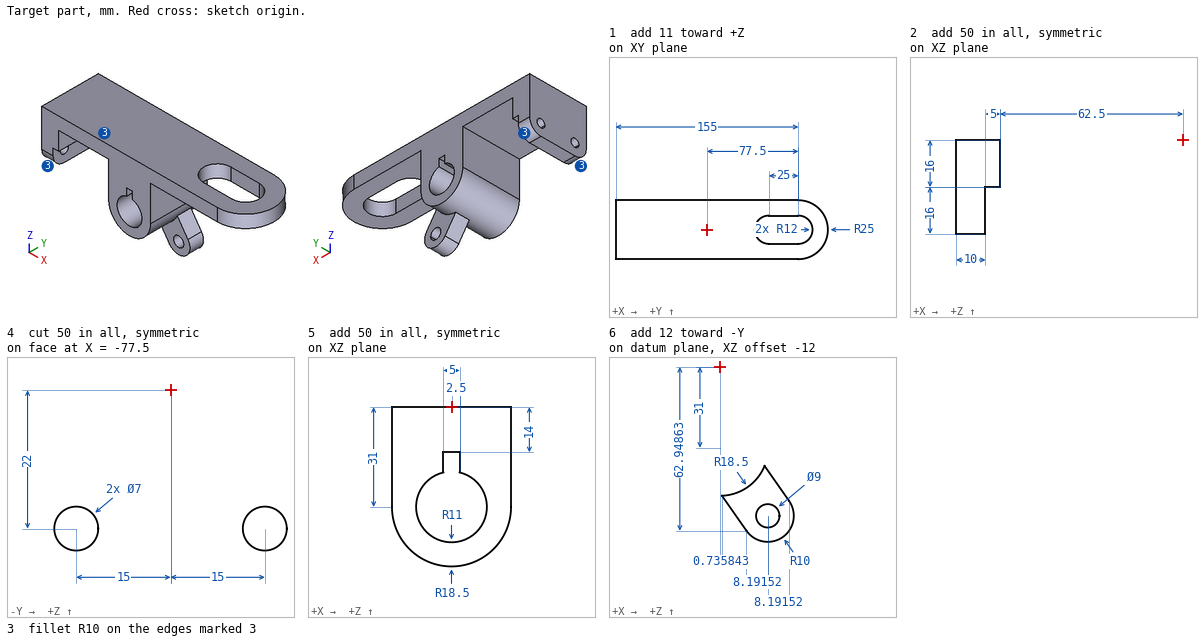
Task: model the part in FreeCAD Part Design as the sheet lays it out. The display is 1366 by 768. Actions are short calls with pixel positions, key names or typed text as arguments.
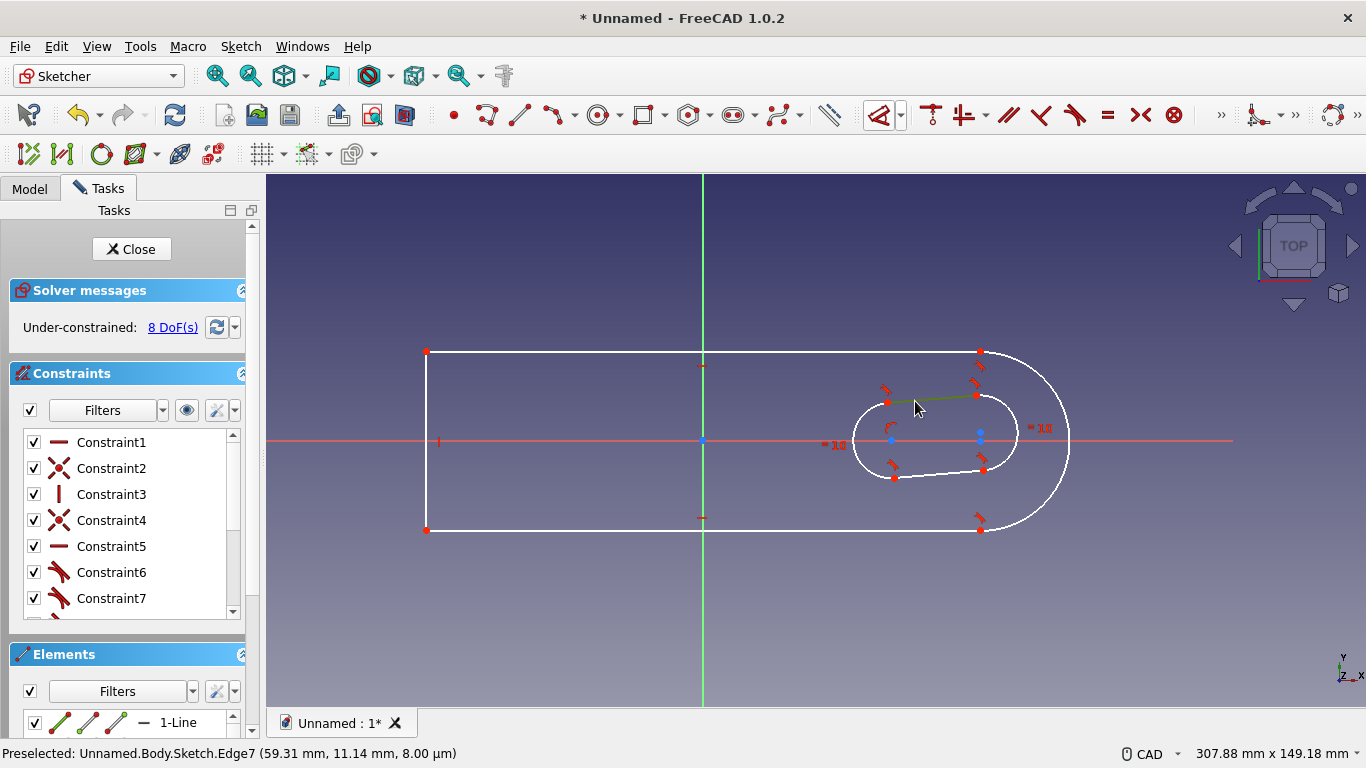
key(h)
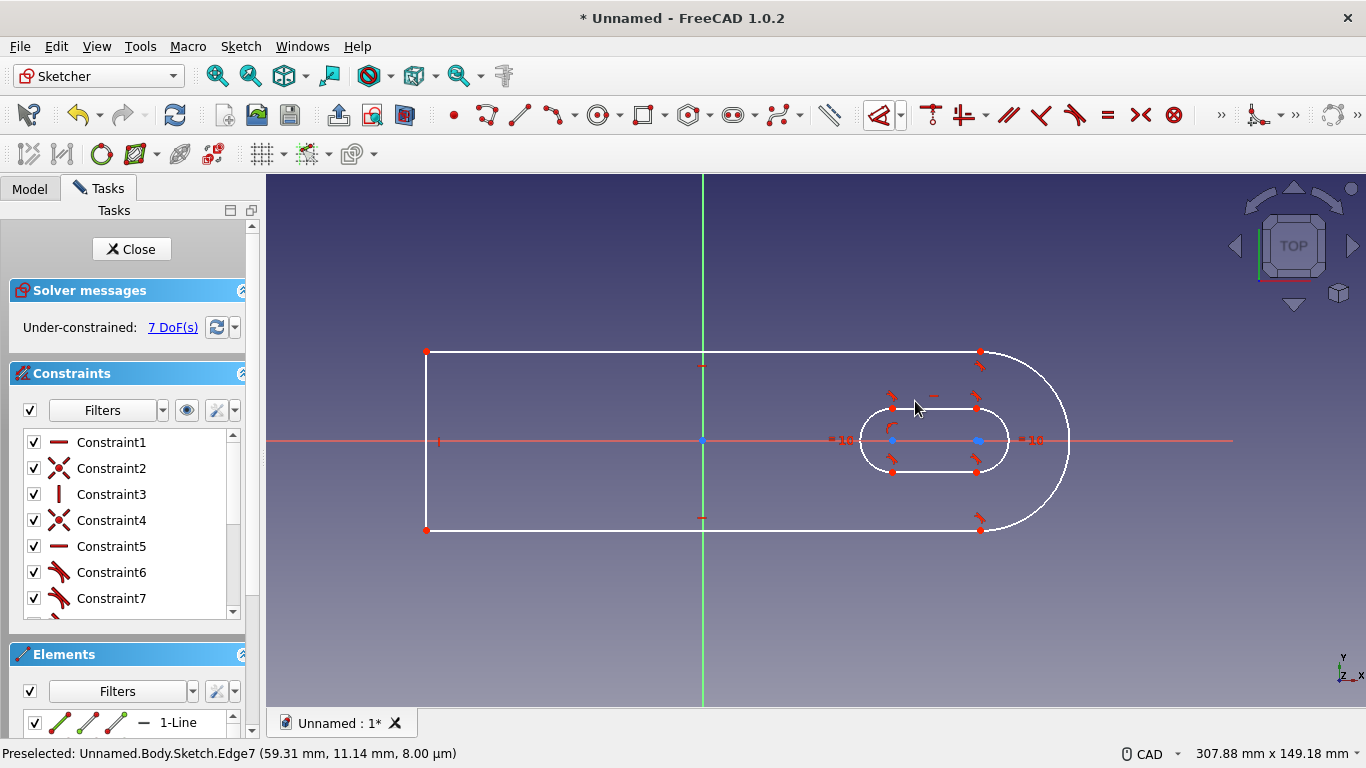
click(1052, 494)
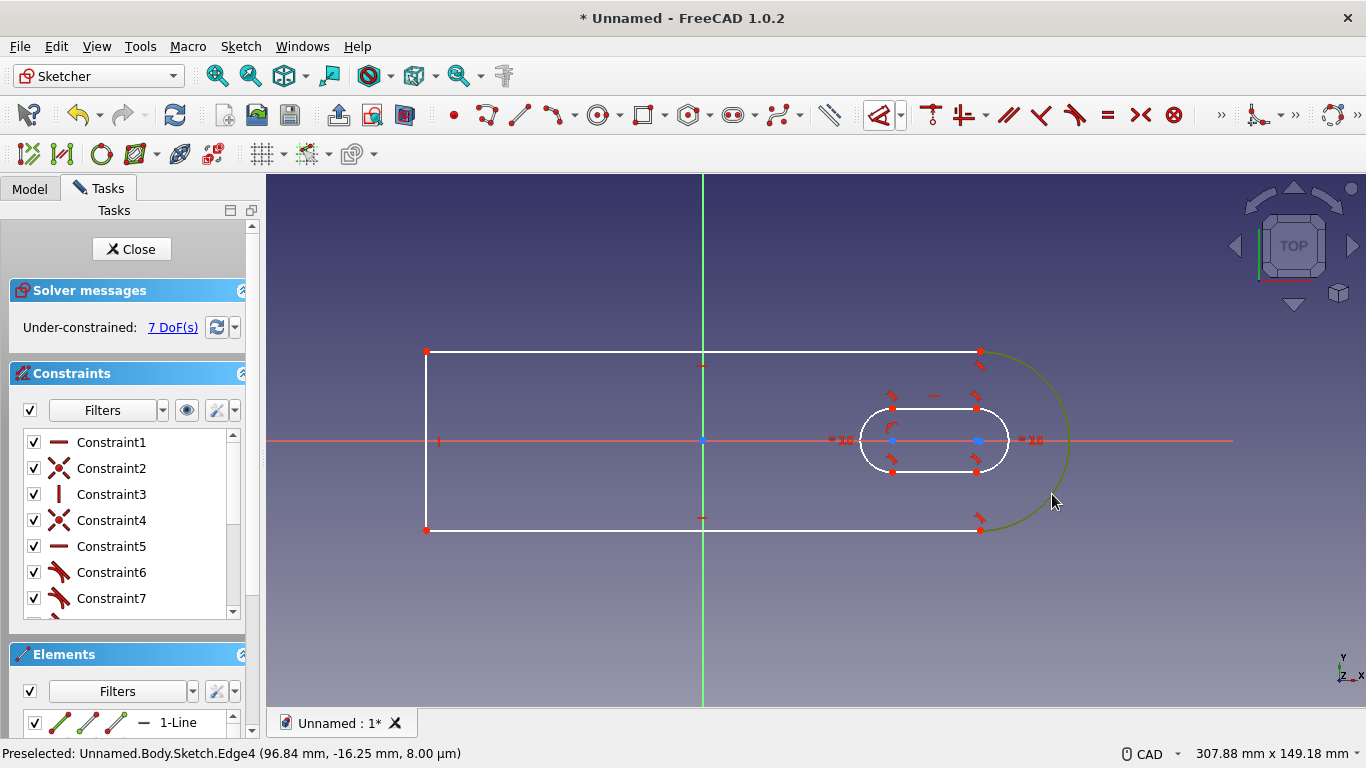
click(1003, 459)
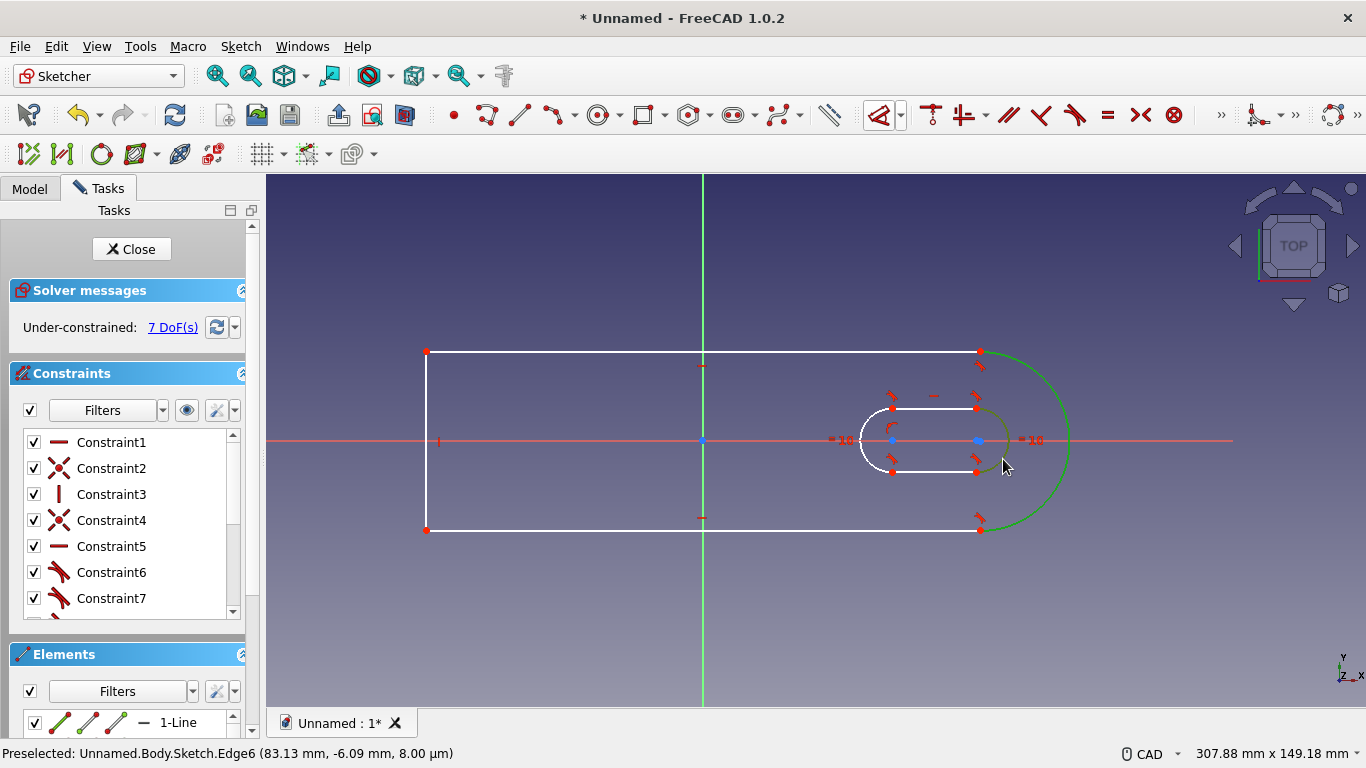
click(931, 116)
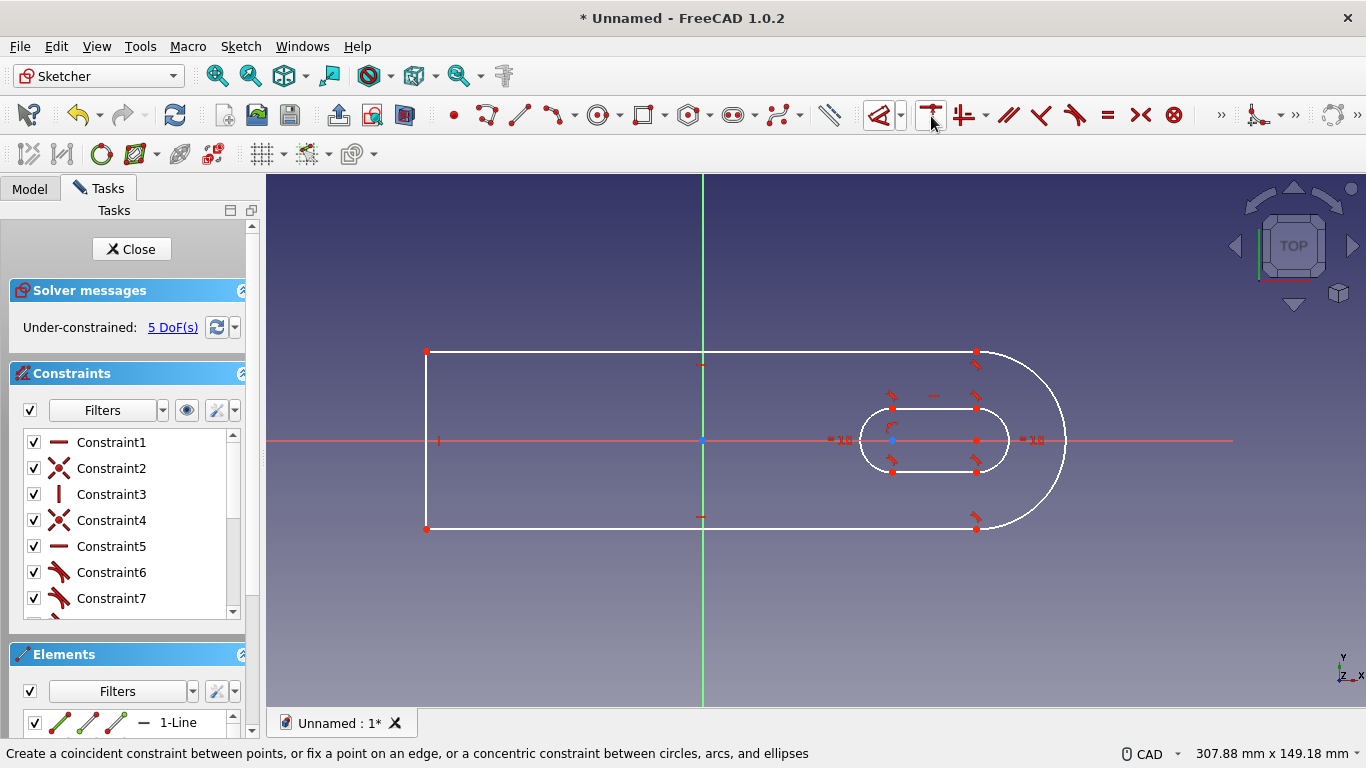
click(878, 116)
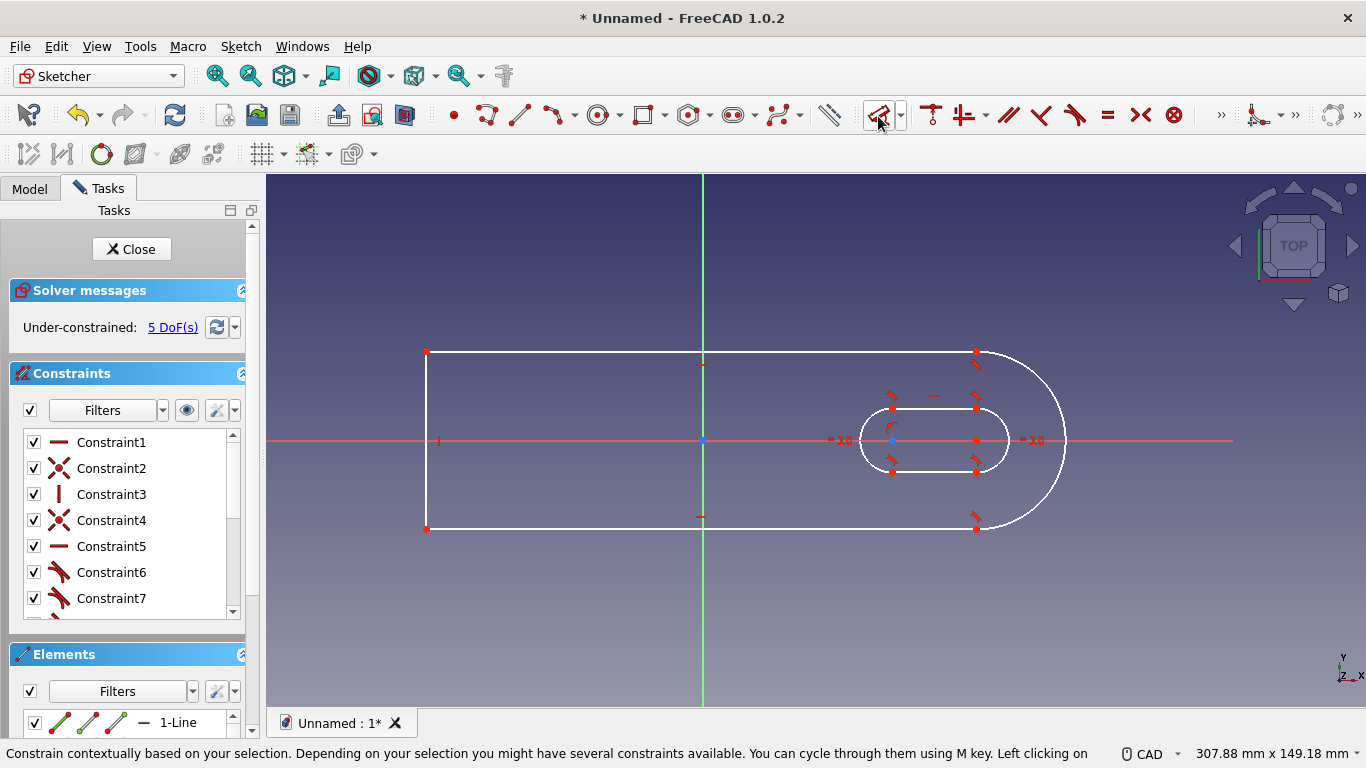
click(1049, 493)
click(1075, 512)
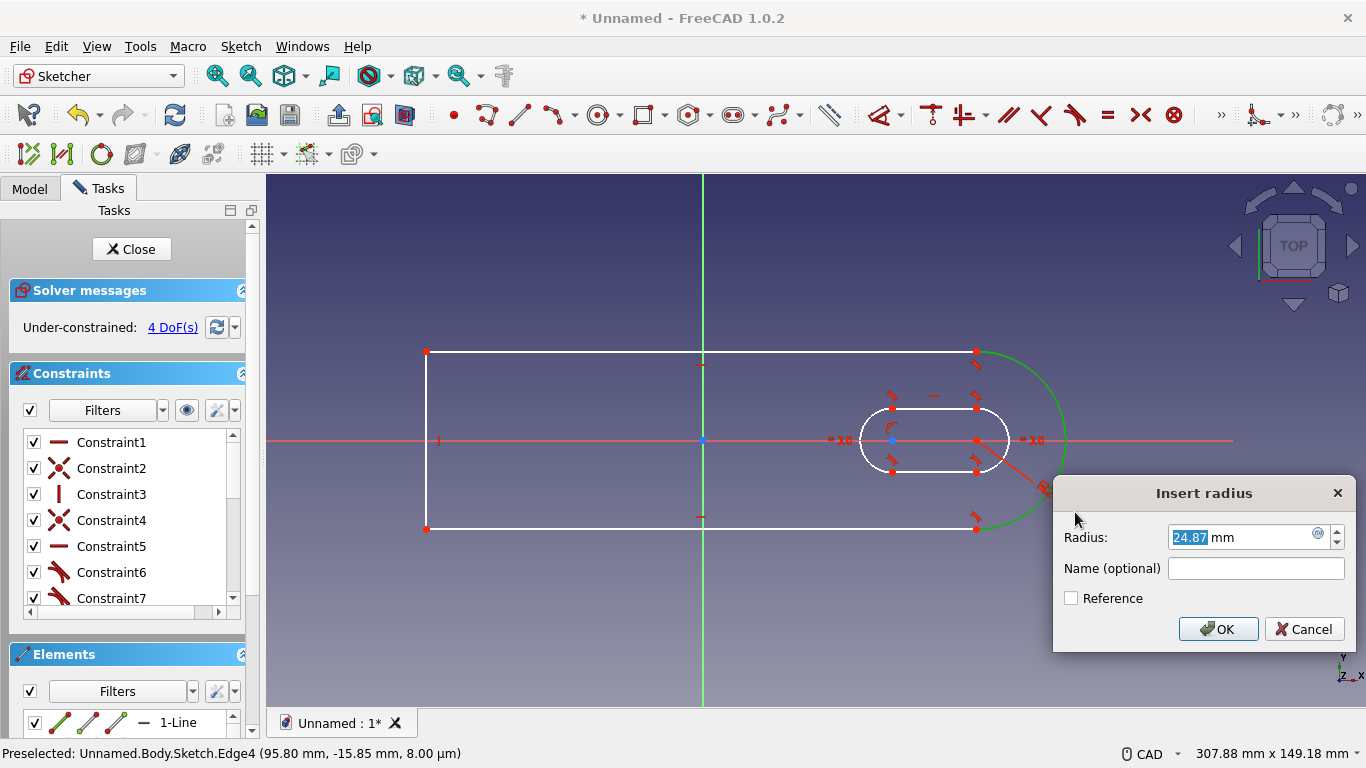
text(25)
key(Return)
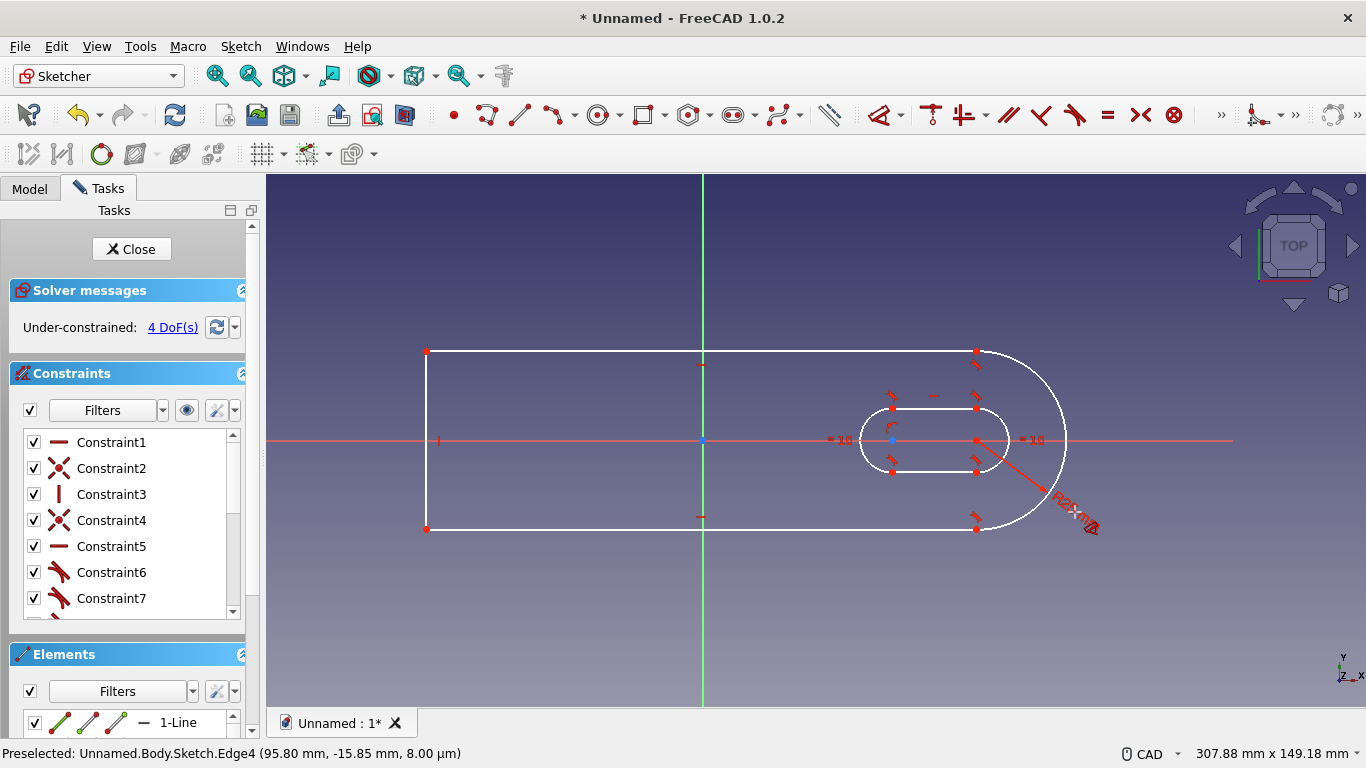
click(866, 422)
click(840, 404)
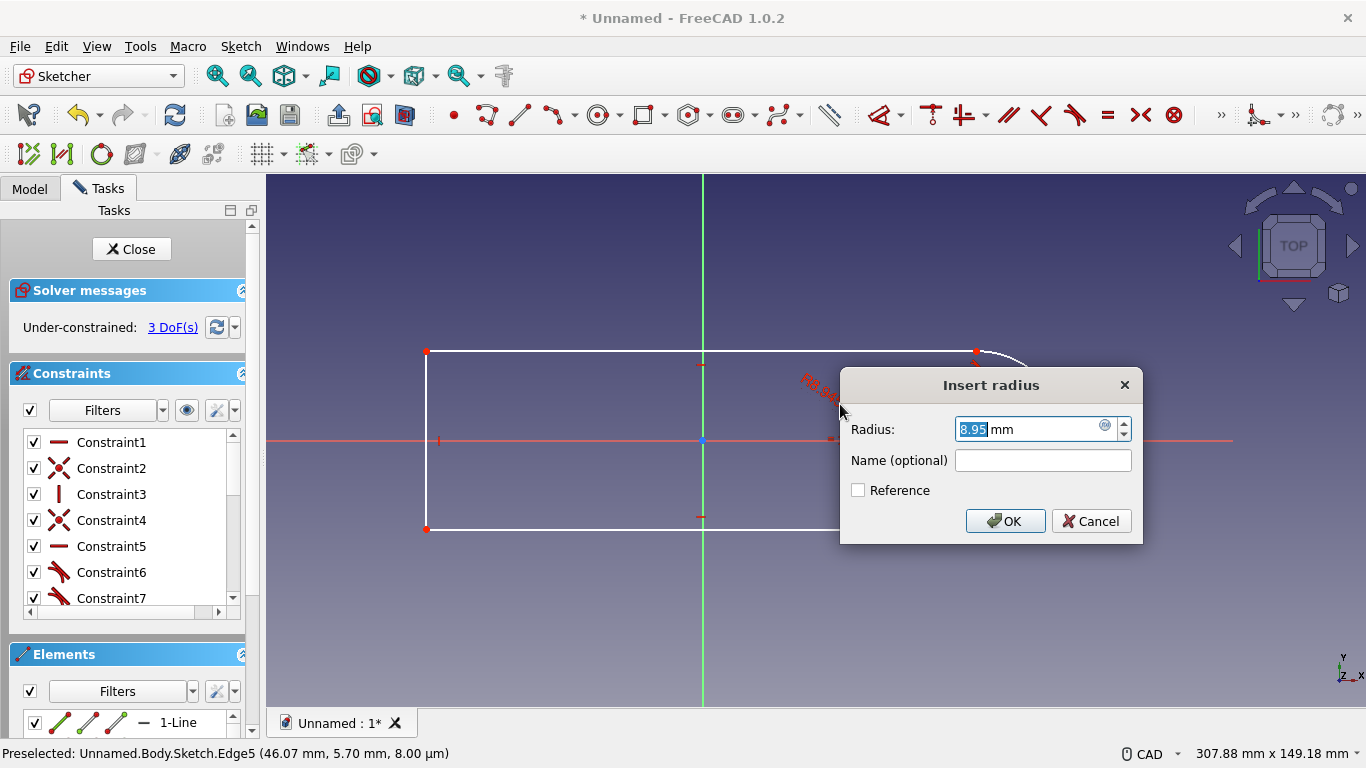
text(12)
key(Return)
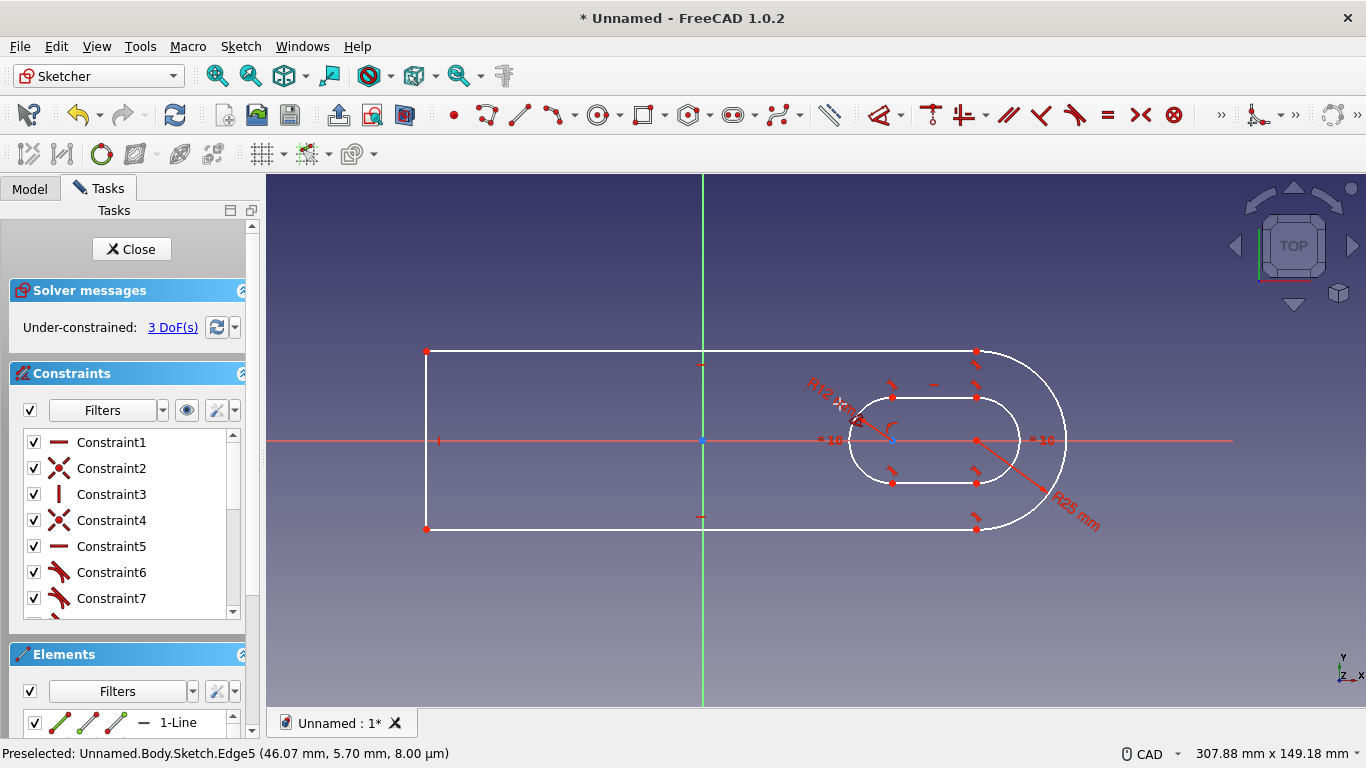
click(918, 398)
click(935, 456)